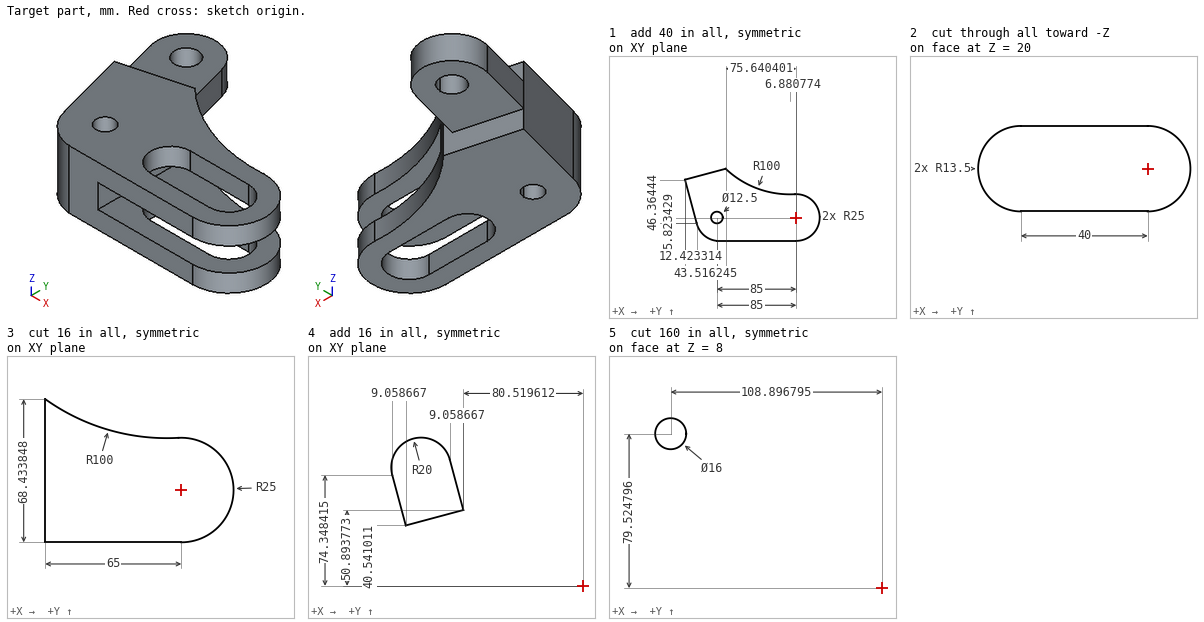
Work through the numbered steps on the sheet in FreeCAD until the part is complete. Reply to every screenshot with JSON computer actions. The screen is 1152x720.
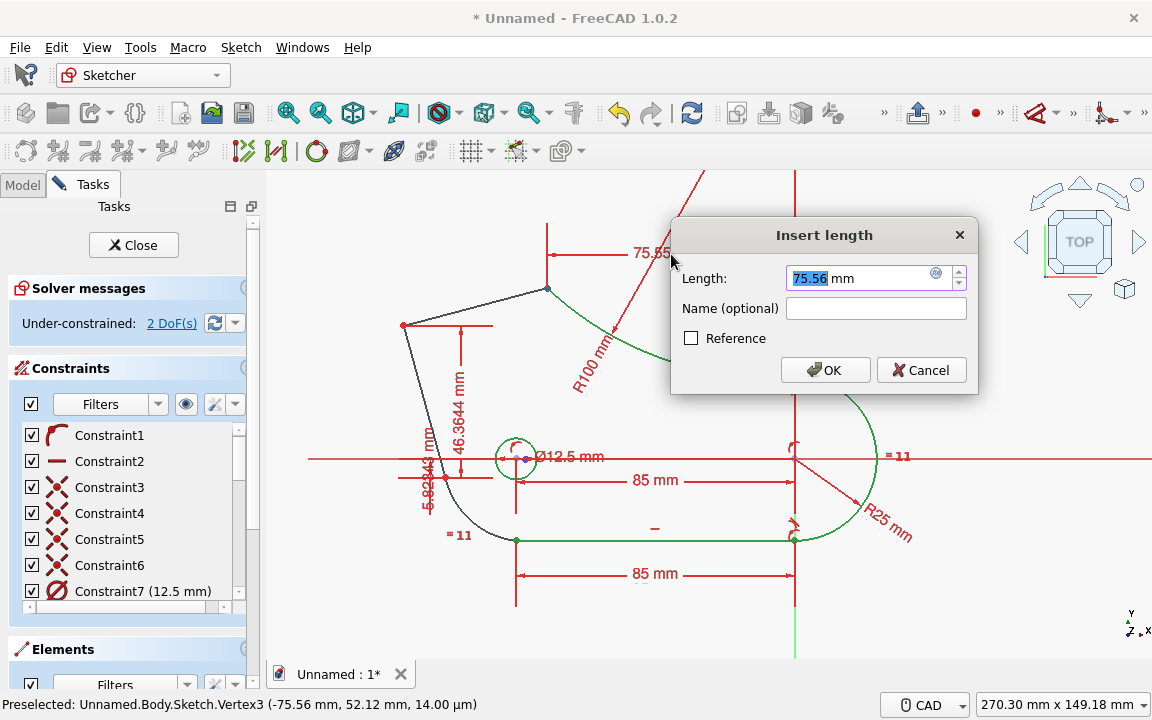
{"action": "type", "text": "75.640401"}
{"action": "key", "text": "Return"}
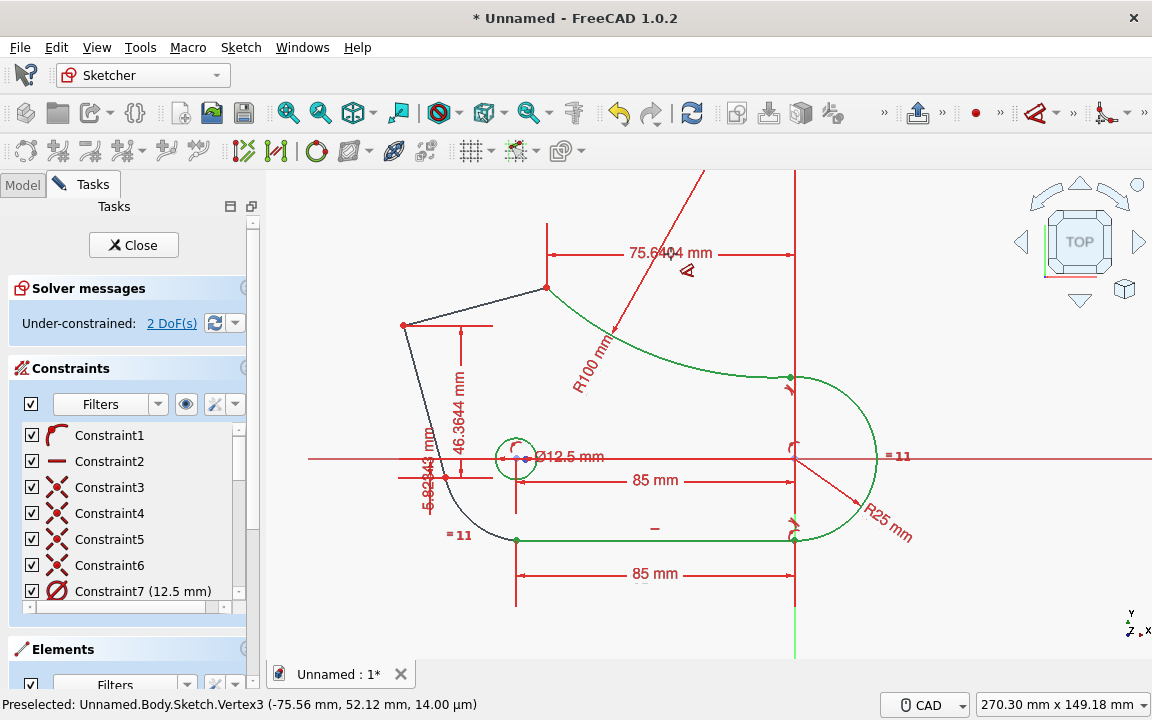
{"action": "left_click", "coordinate": [504, 299]}
{"action": "left_click", "coordinate": [475, 254]}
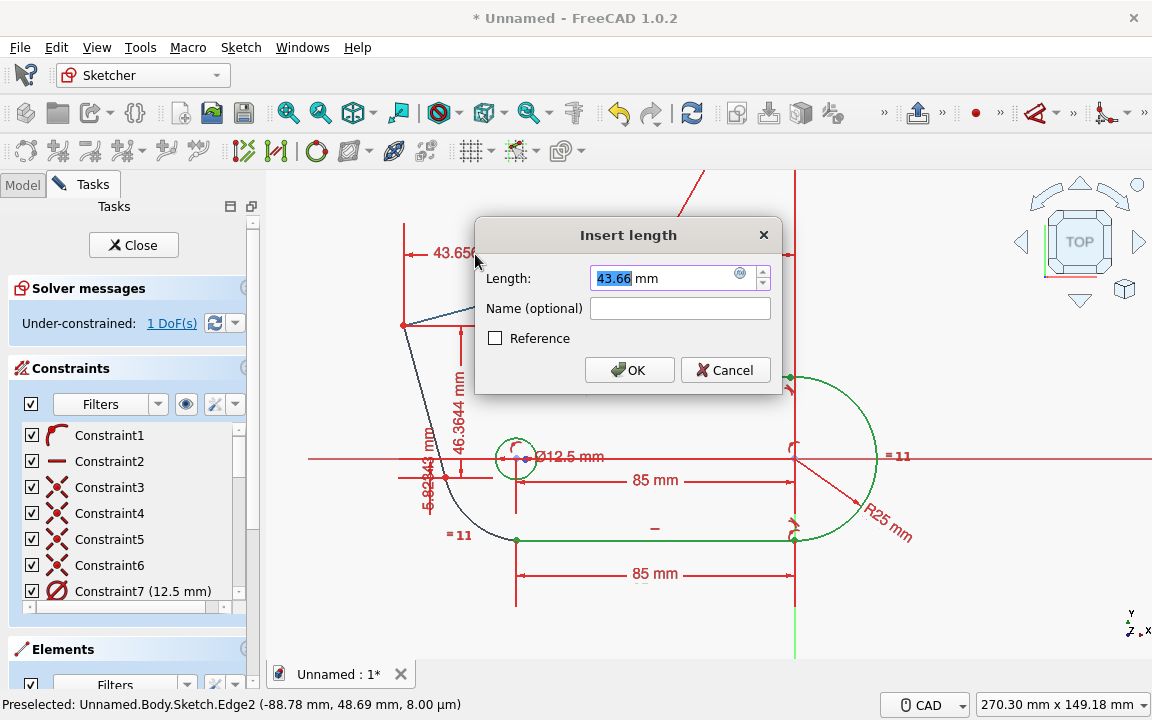
{"action": "type", "text": "43.516245"}
{"action": "key", "text": "Return"}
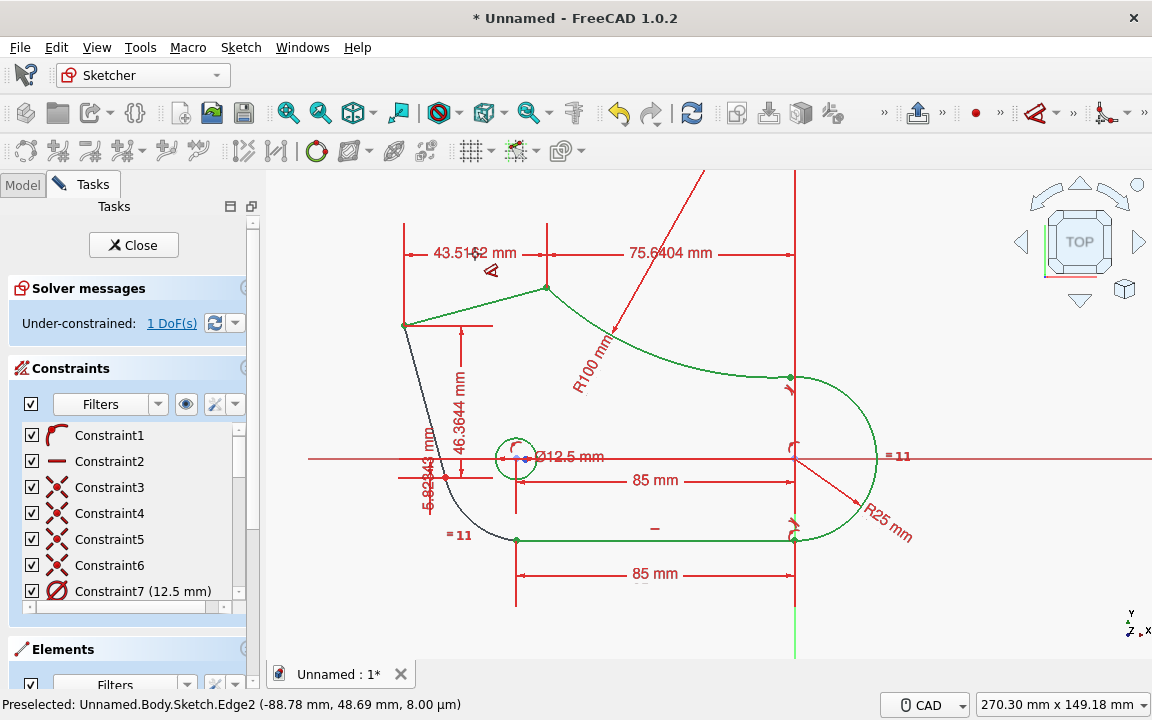
{"action": "left_click", "coordinate": [417, 372]}
{"action": "left_click", "coordinate": [425, 292]}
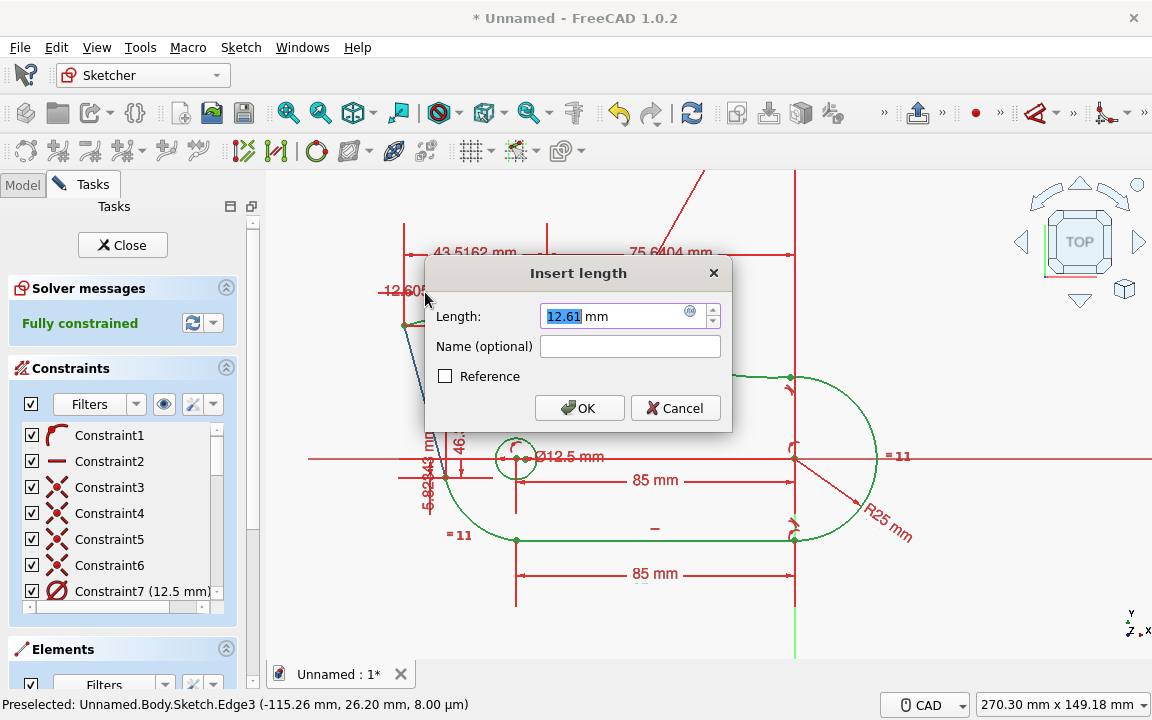
{"action": "type", "text": "12.423314"}
{"action": "key", "text": "Return"}
{"action": "key", "text": "Escape"}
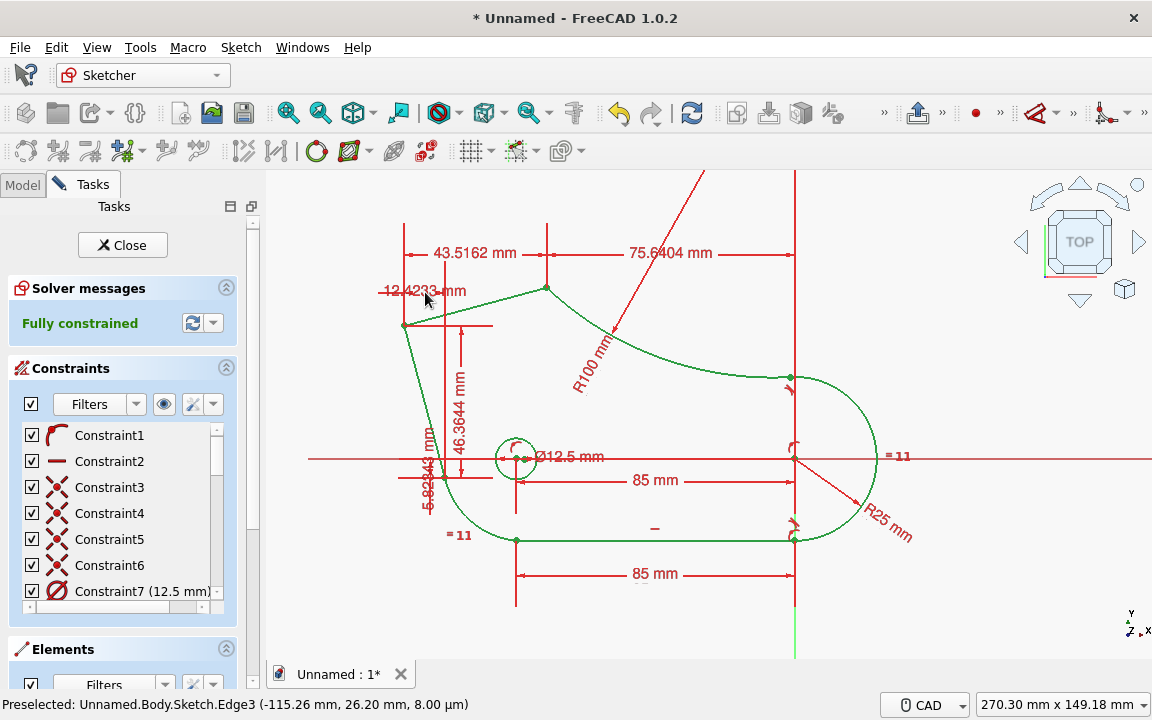
{"action": "left_click", "coordinate": [123, 245]}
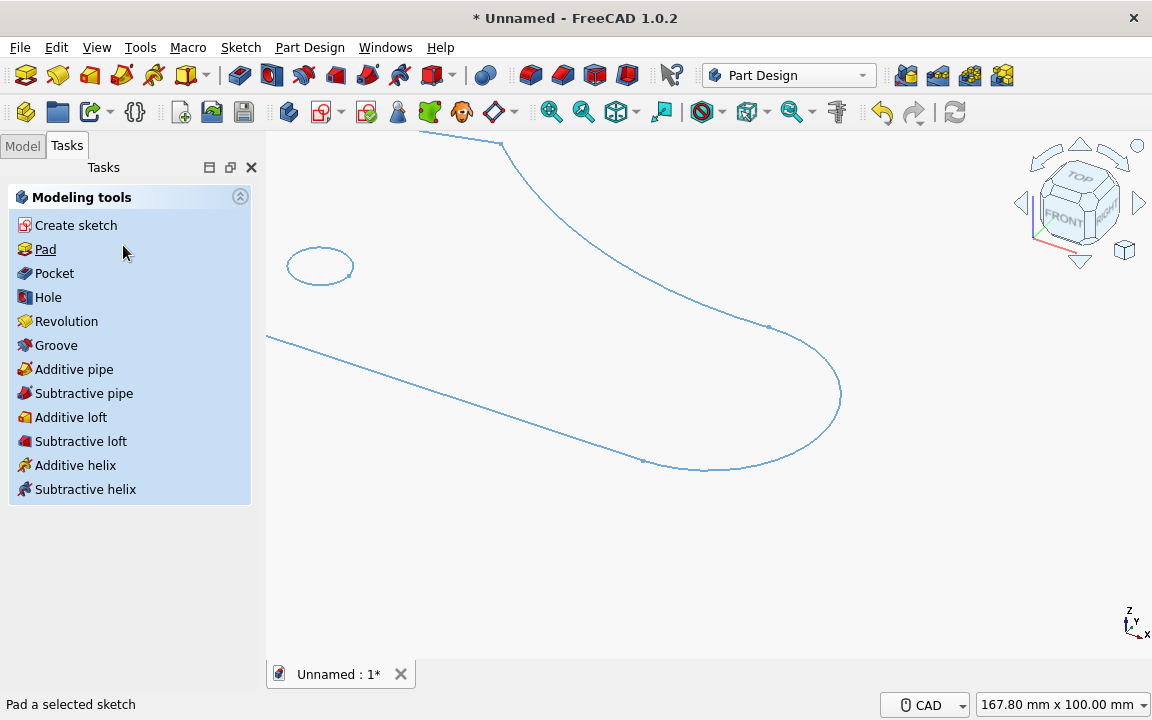
{"action": "left_click", "coordinate": [26, 76]}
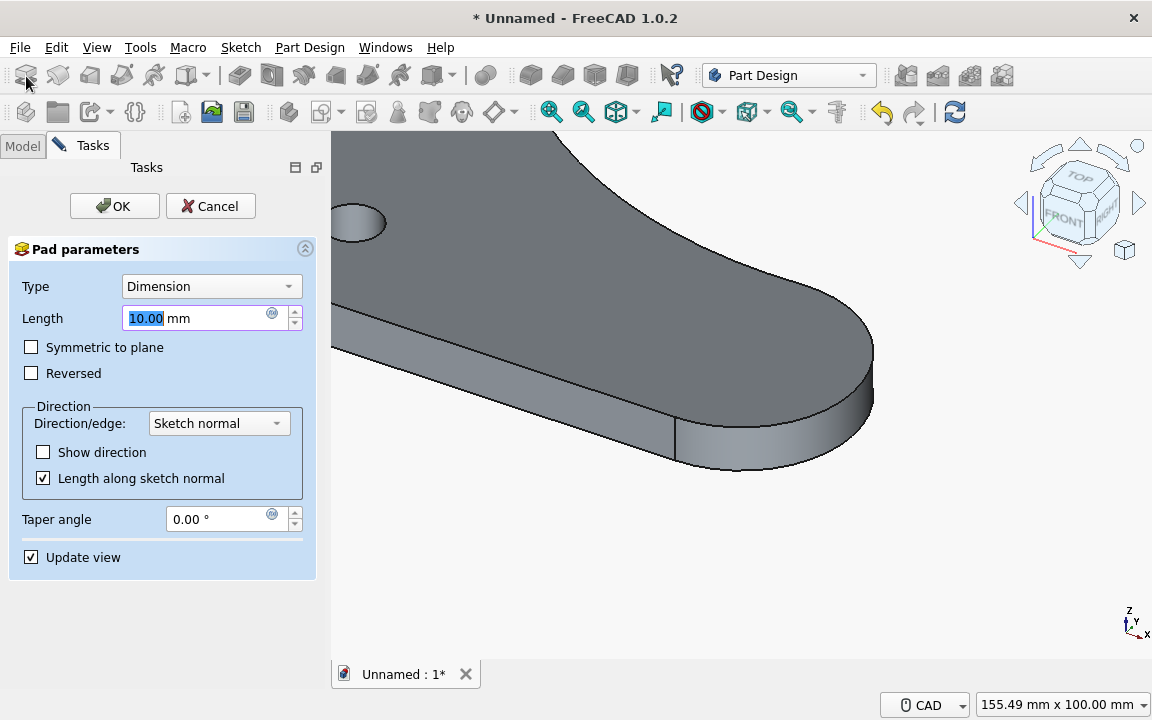
{"action": "type", "text": "40"}
{"action": "key", "text": "Tab"}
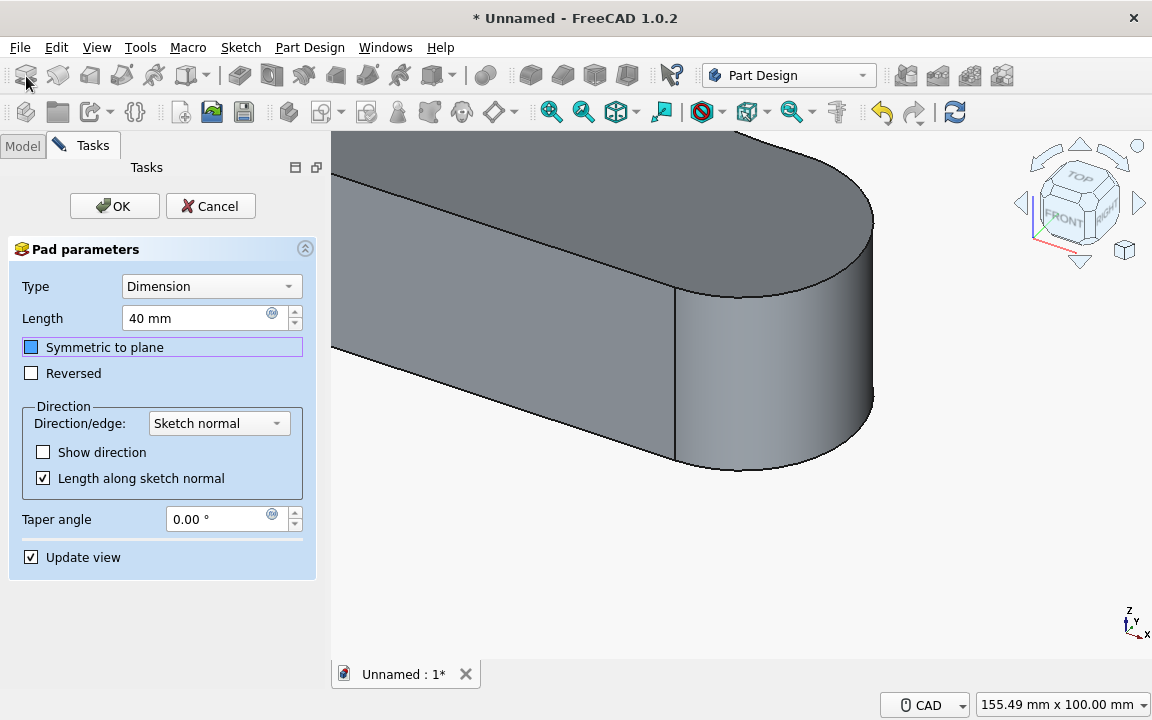
{"action": "left_click", "coordinate": [30, 347]}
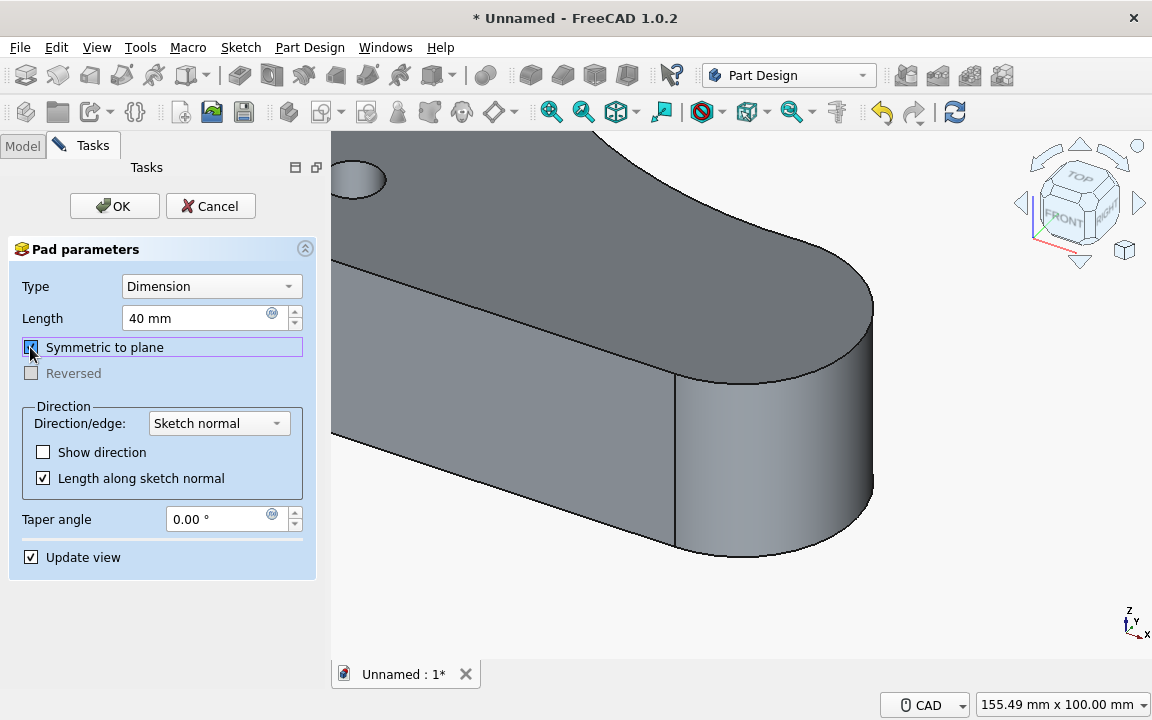
{"action": "left_click", "coordinate": [115, 206]}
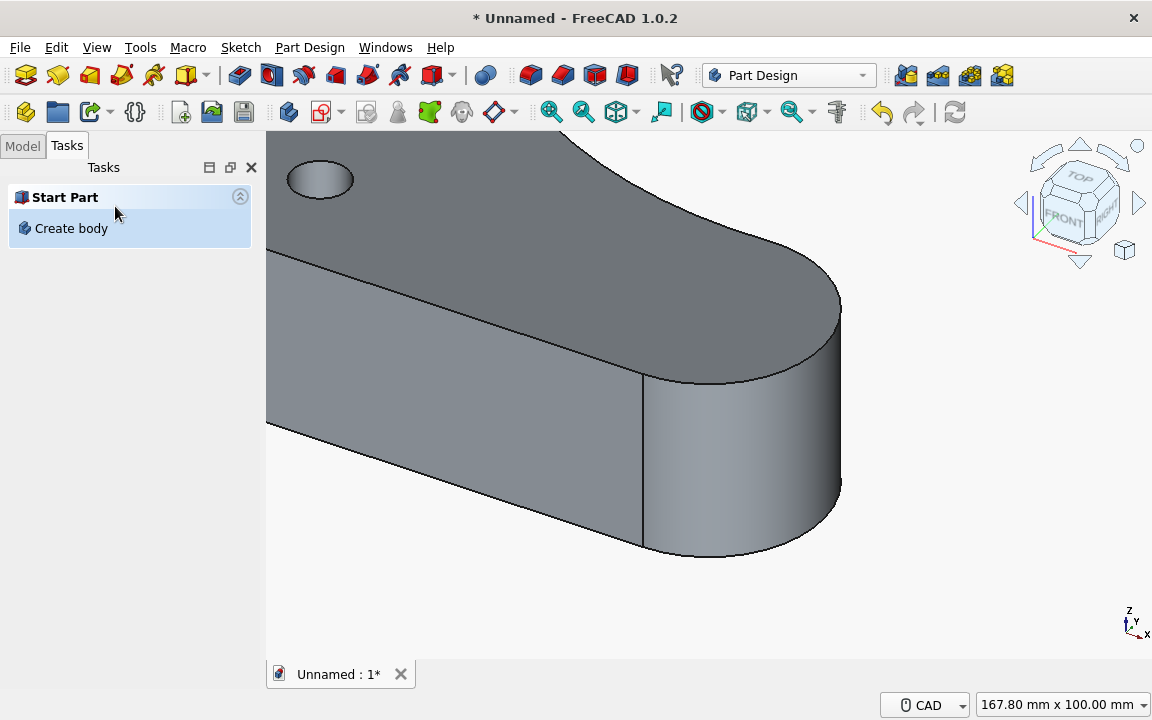
{"action": "left_click", "coordinate": [552, 112]}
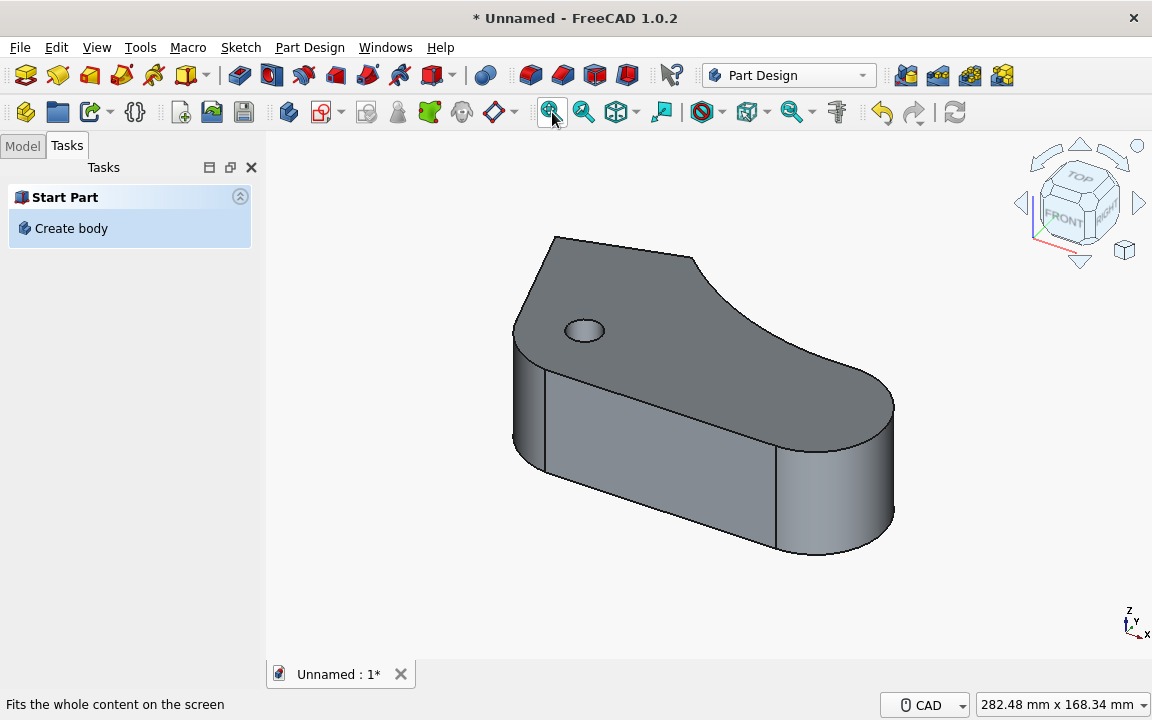
{"action": "left_click", "coordinate": [692, 360]}